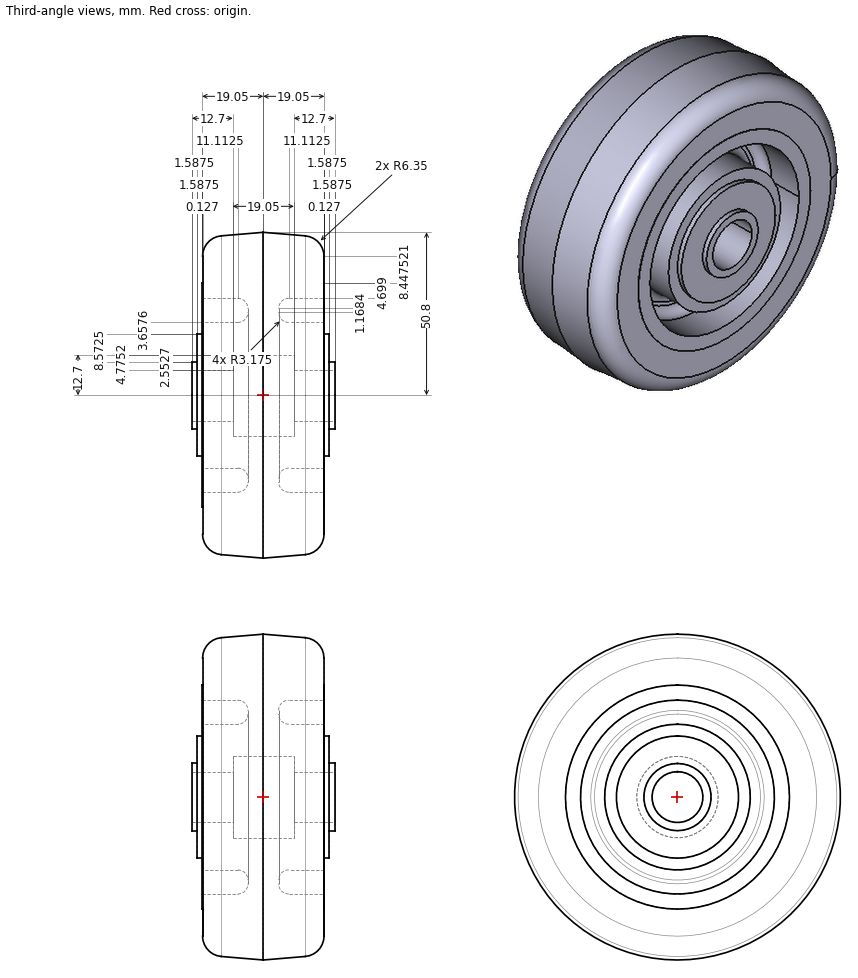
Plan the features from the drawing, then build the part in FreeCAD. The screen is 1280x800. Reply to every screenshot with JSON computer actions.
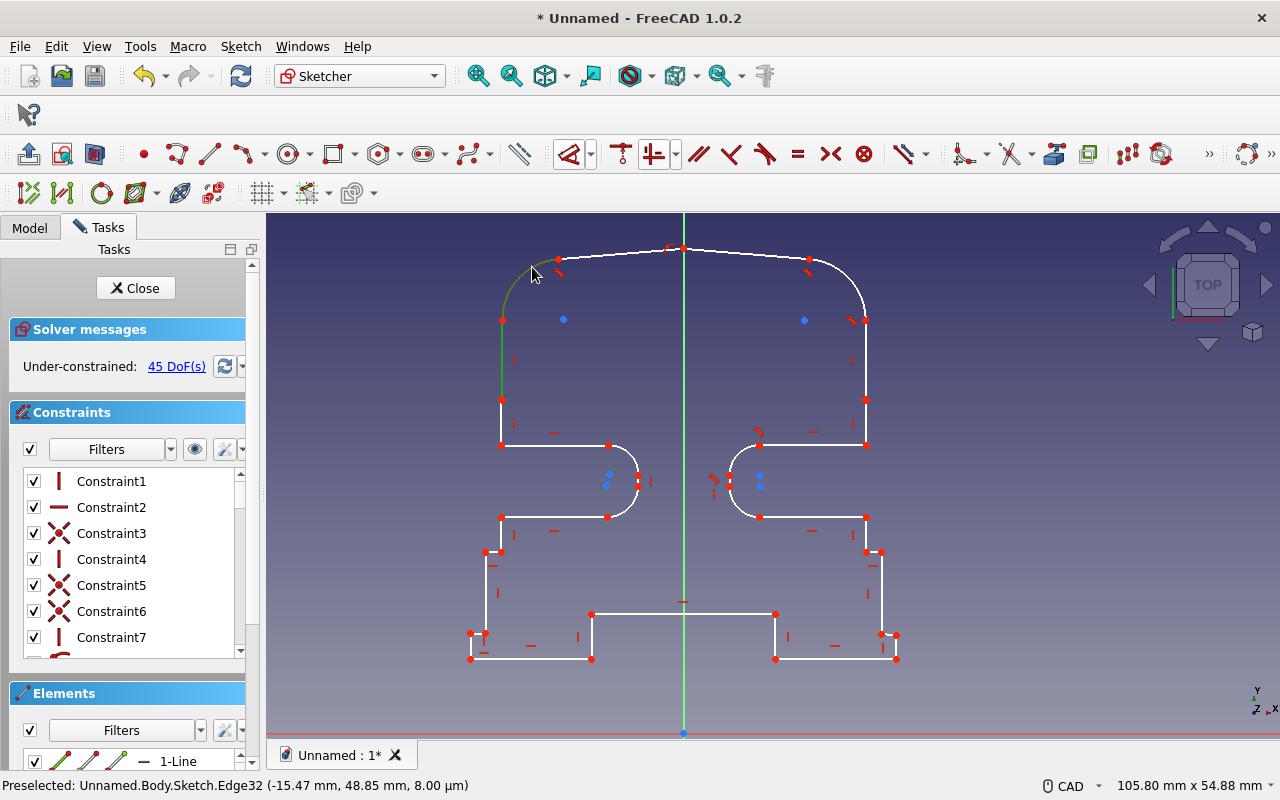
{"action": "left_click", "coordinate": [765, 154]}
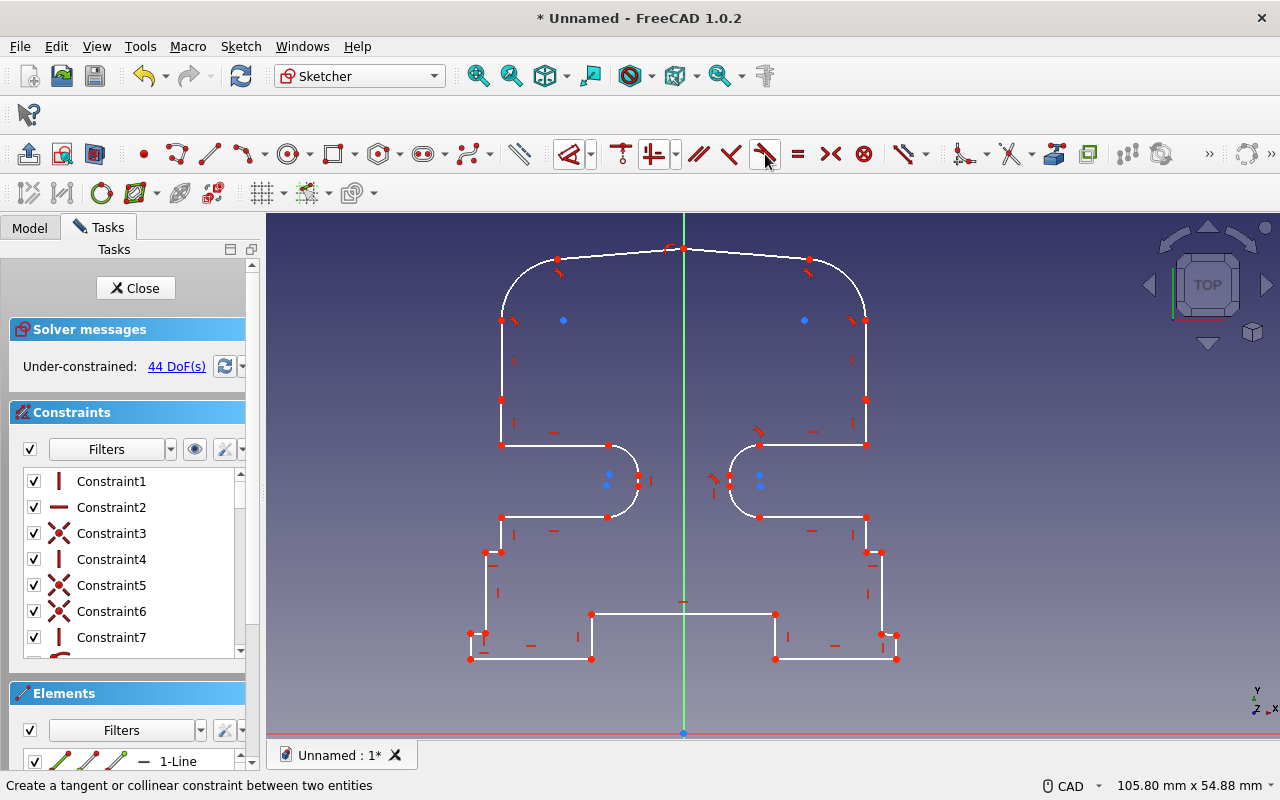
{"action": "left_click", "coordinate": [533, 446]}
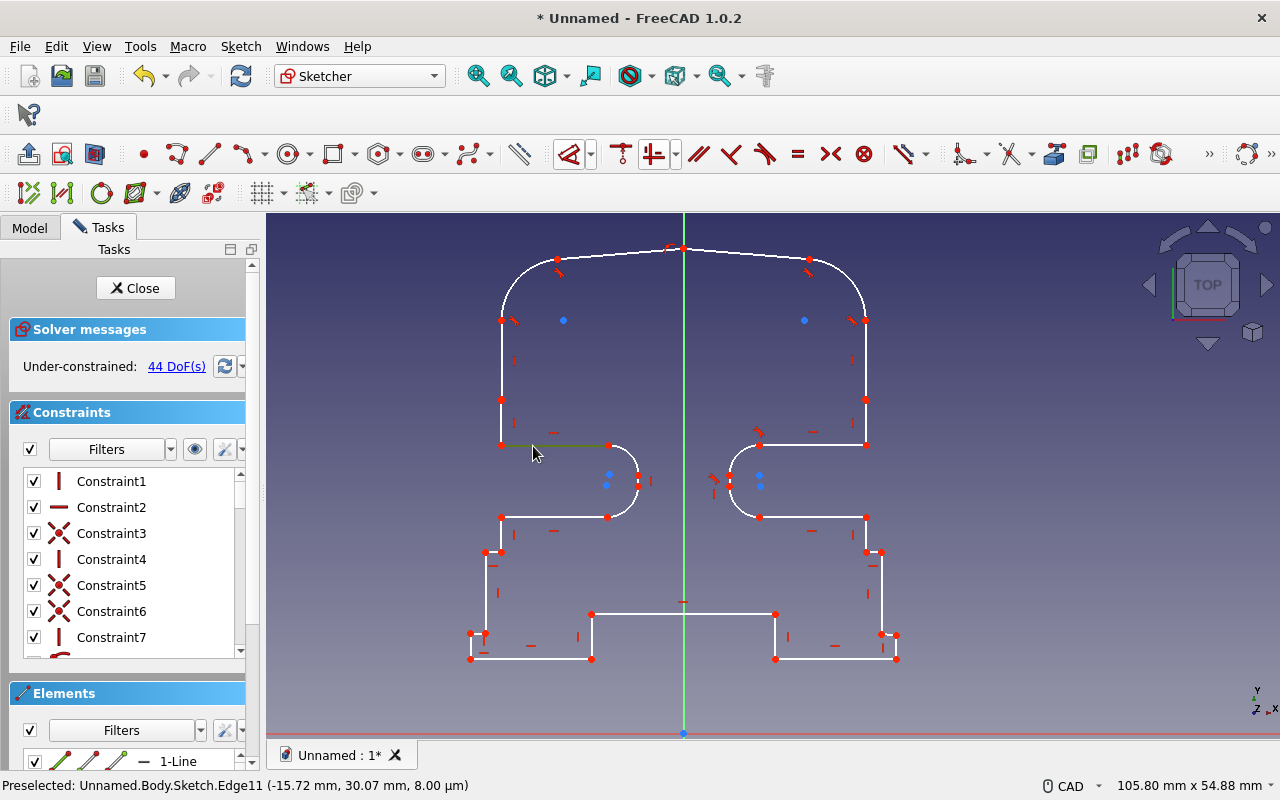
{"action": "left_click", "coordinate": [635, 462]}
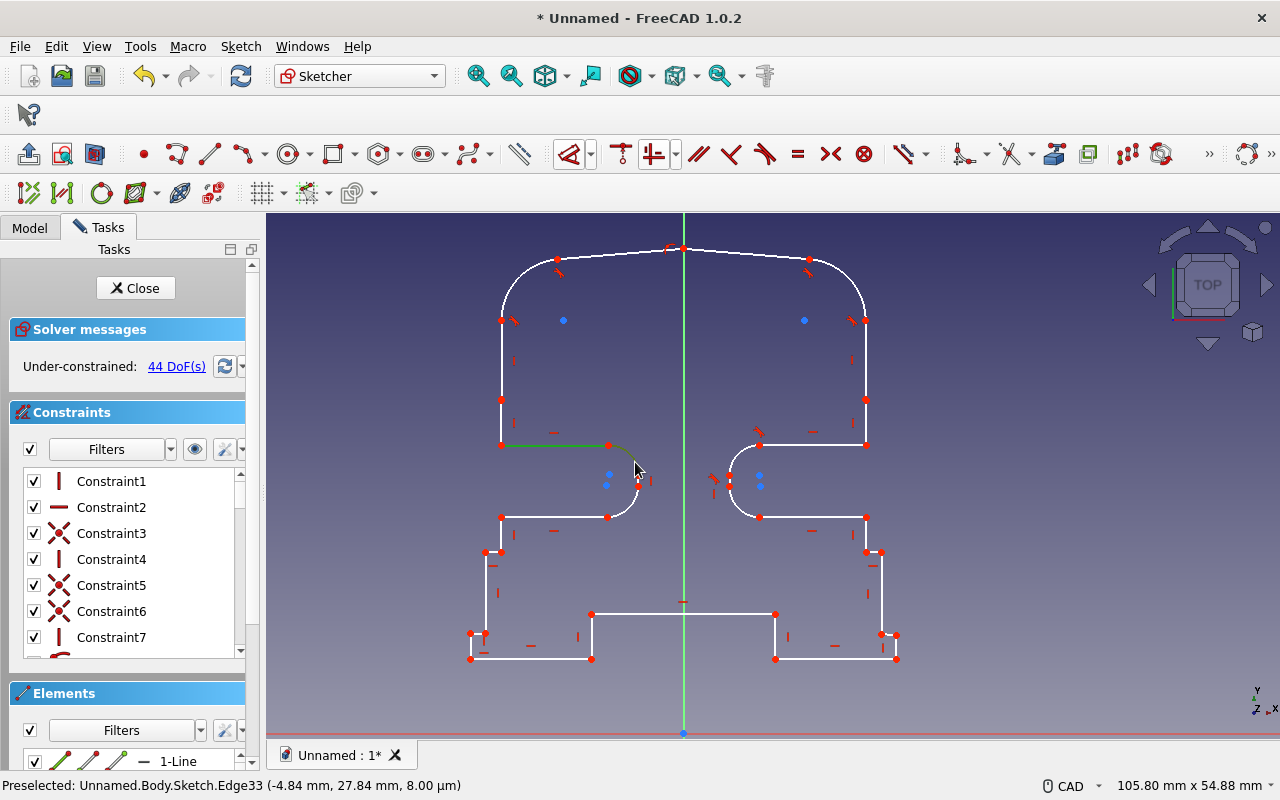
{"action": "left_click", "coordinate": [765, 154]}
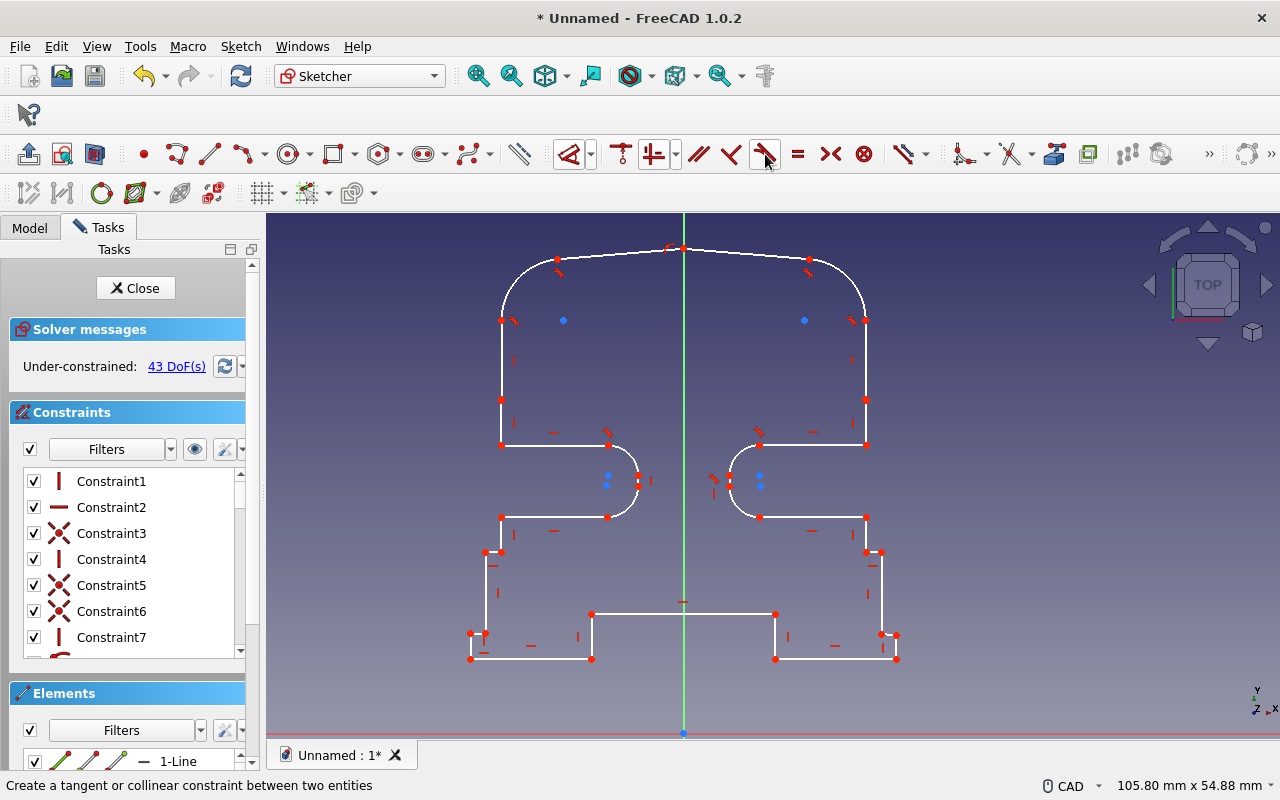
{"action": "scroll", "coordinate": [638, 481], "scroll_direction": "up", "scroll_amount": 5}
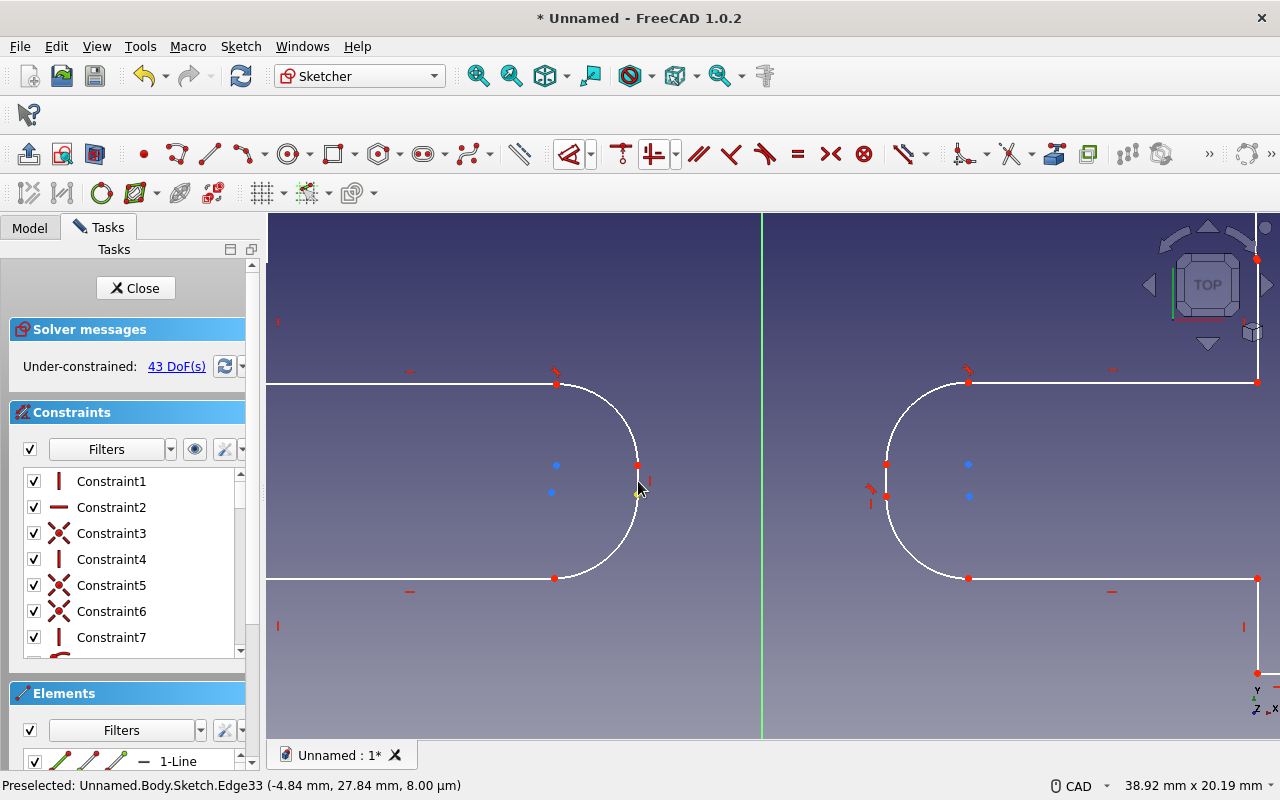
{"action": "left_click", "coordinate": [638, 480]}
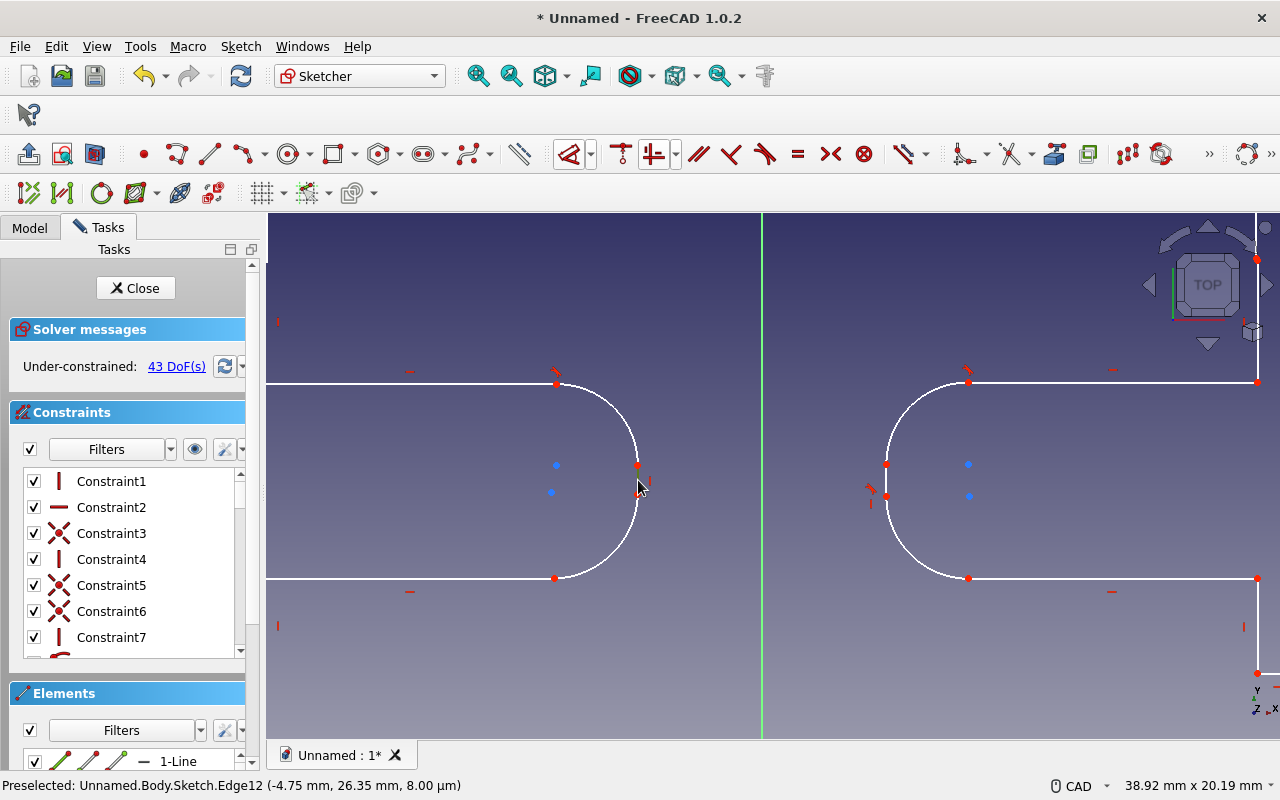
{"action": "left_click", "coordinate": [629, 428]}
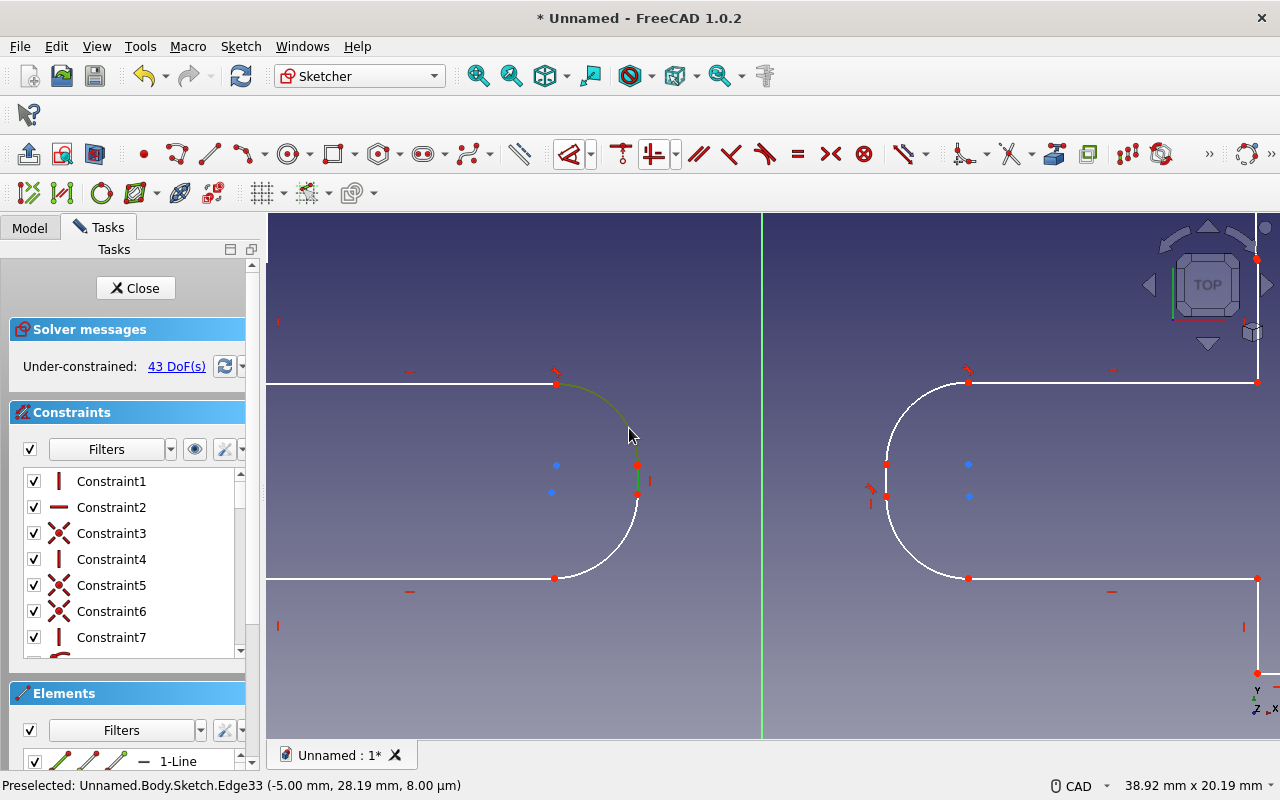
{"action": "left_click", "coordinate": [765, 154]}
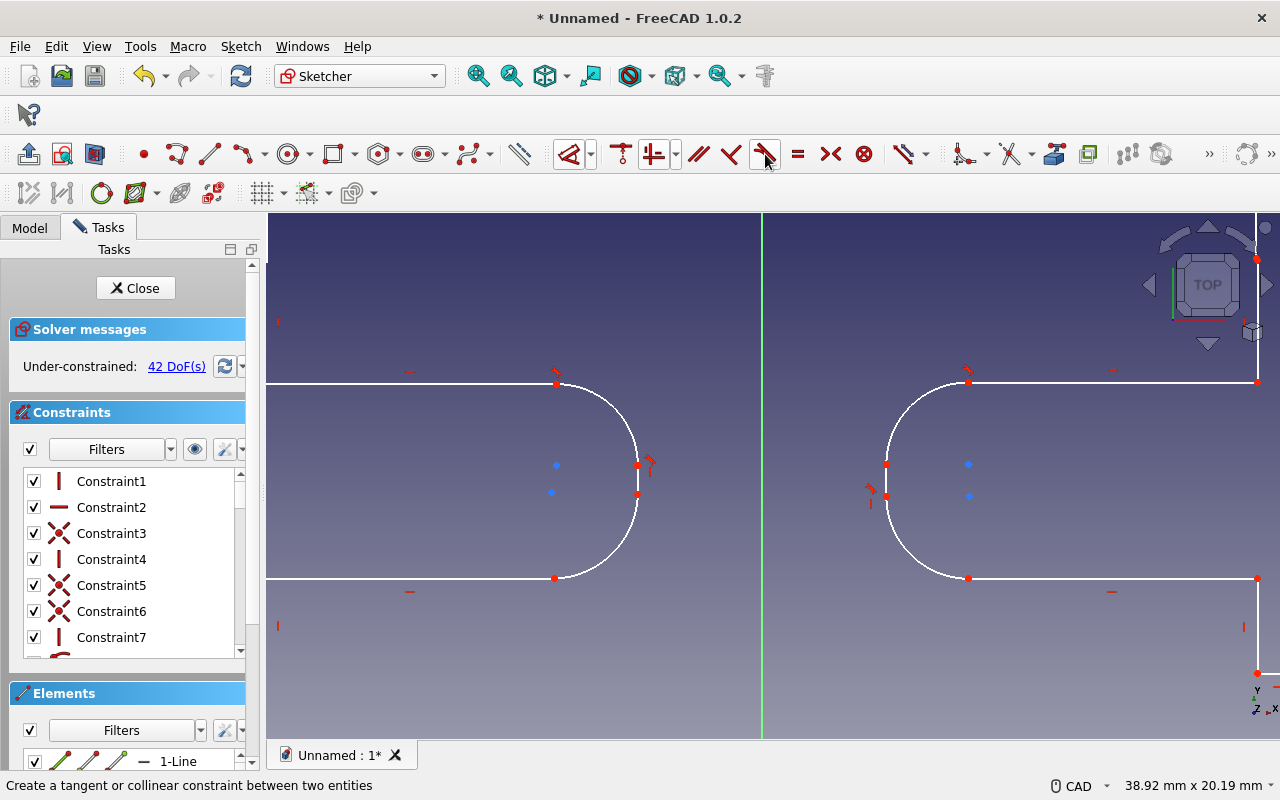
{"action": "left_click", "coordinate": [638, 477]}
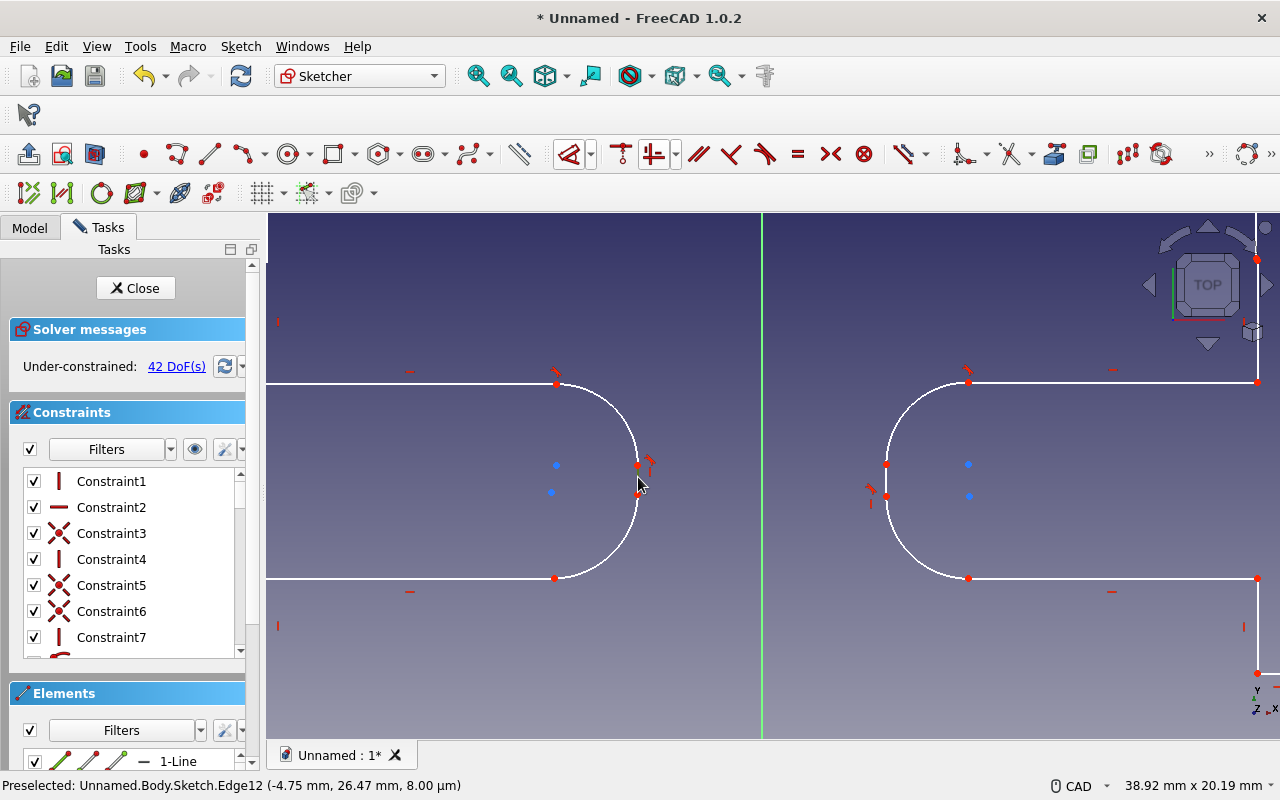
{"action": "left_click", "coordinate": [592, 568]}